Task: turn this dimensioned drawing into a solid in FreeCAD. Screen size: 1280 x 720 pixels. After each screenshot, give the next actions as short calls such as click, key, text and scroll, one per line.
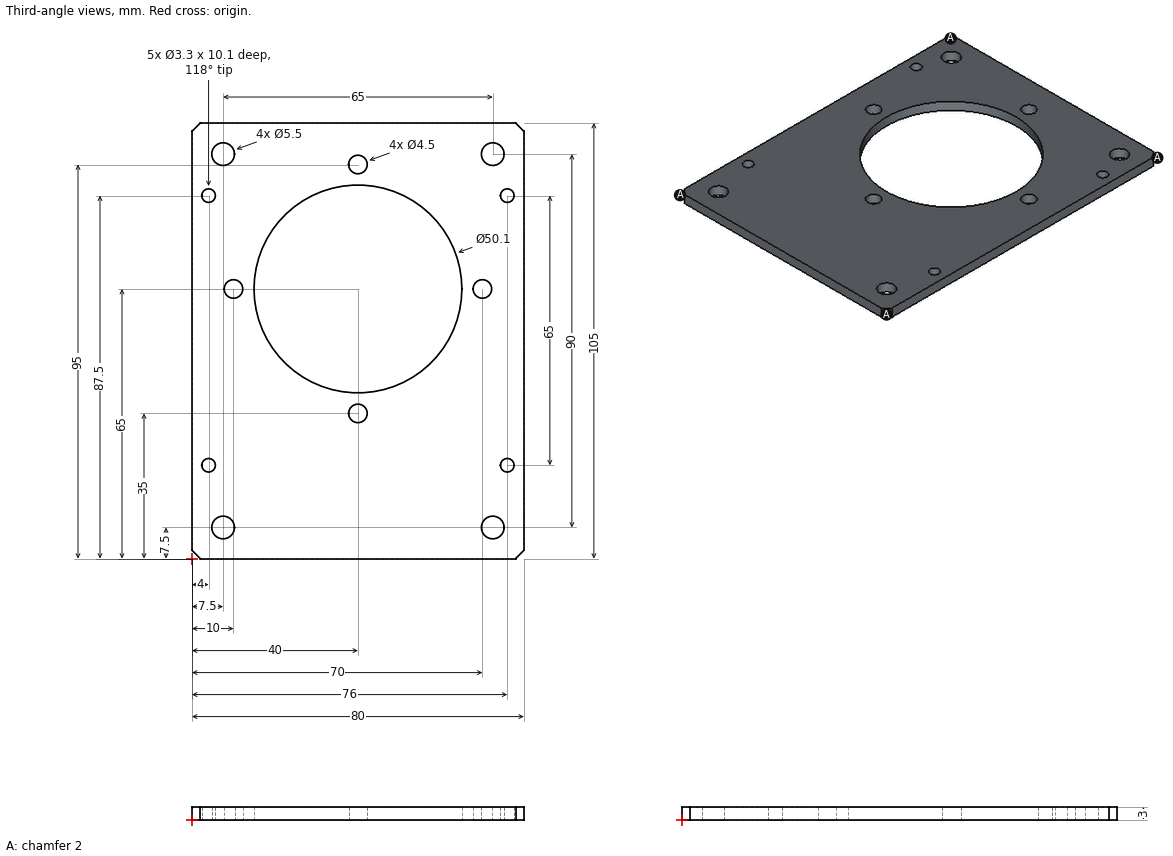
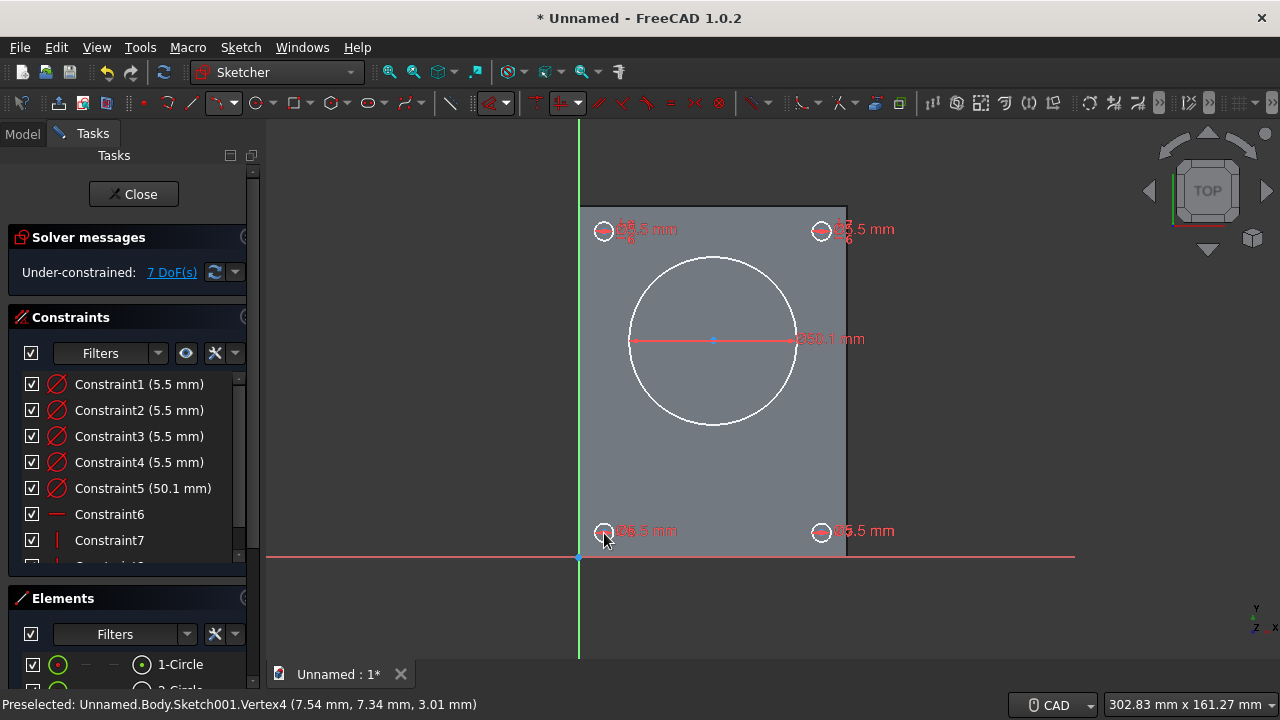
click(822, 533)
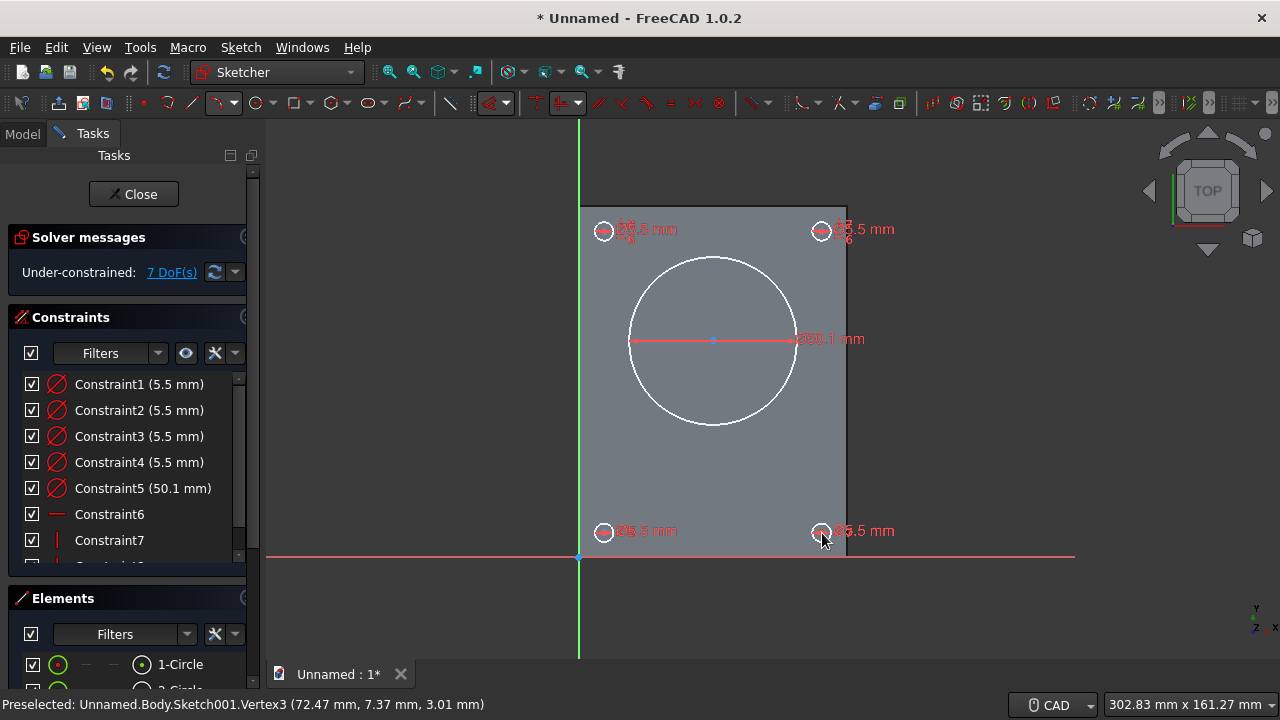
click(604, 533)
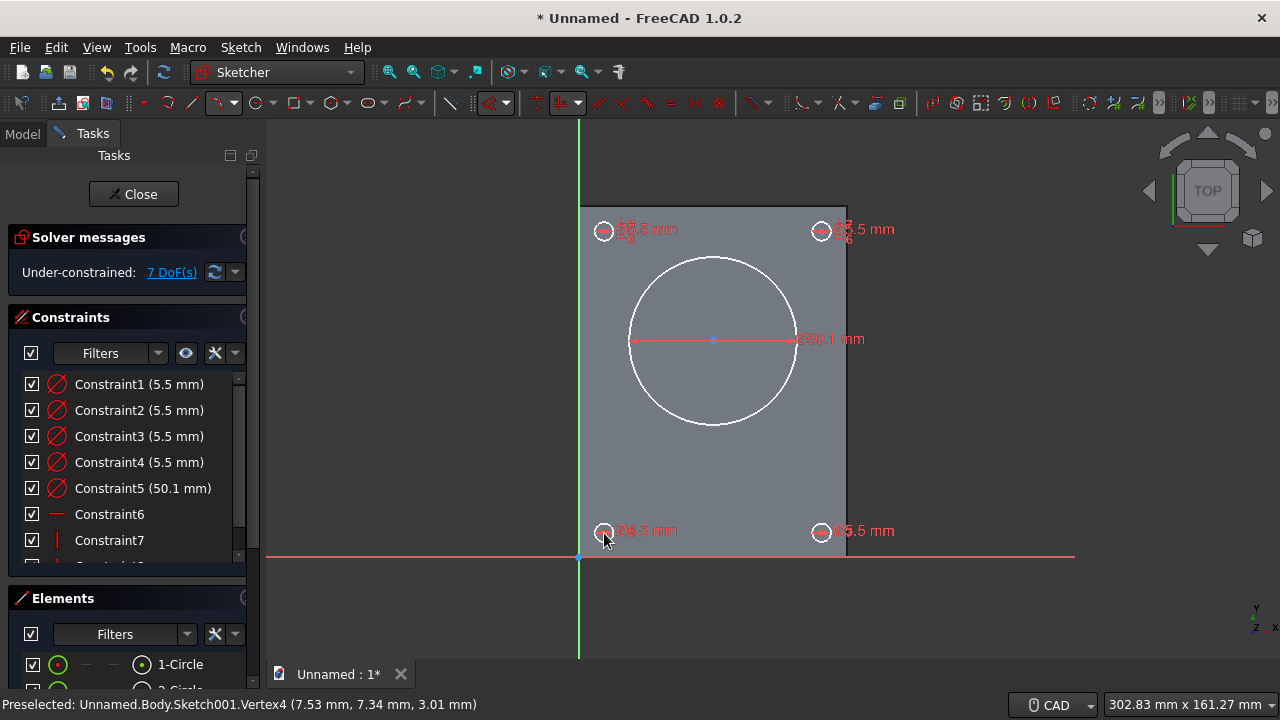
click(580, 104)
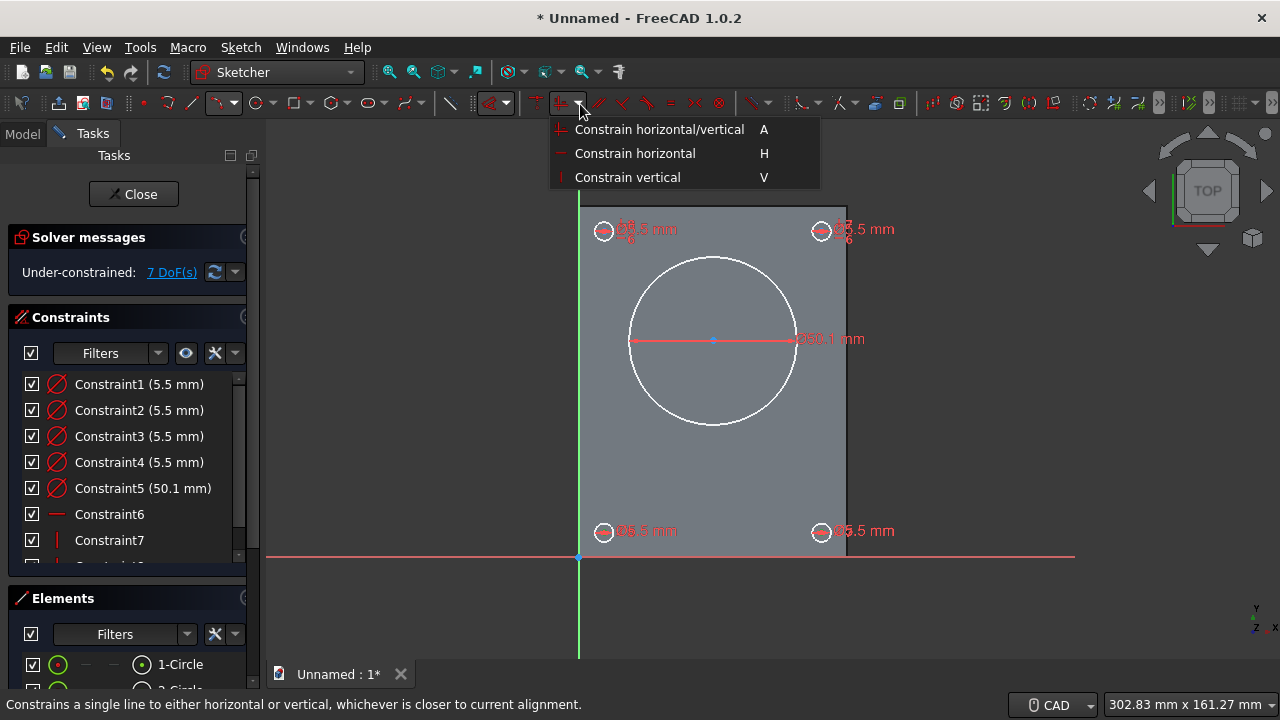
click(685, 153)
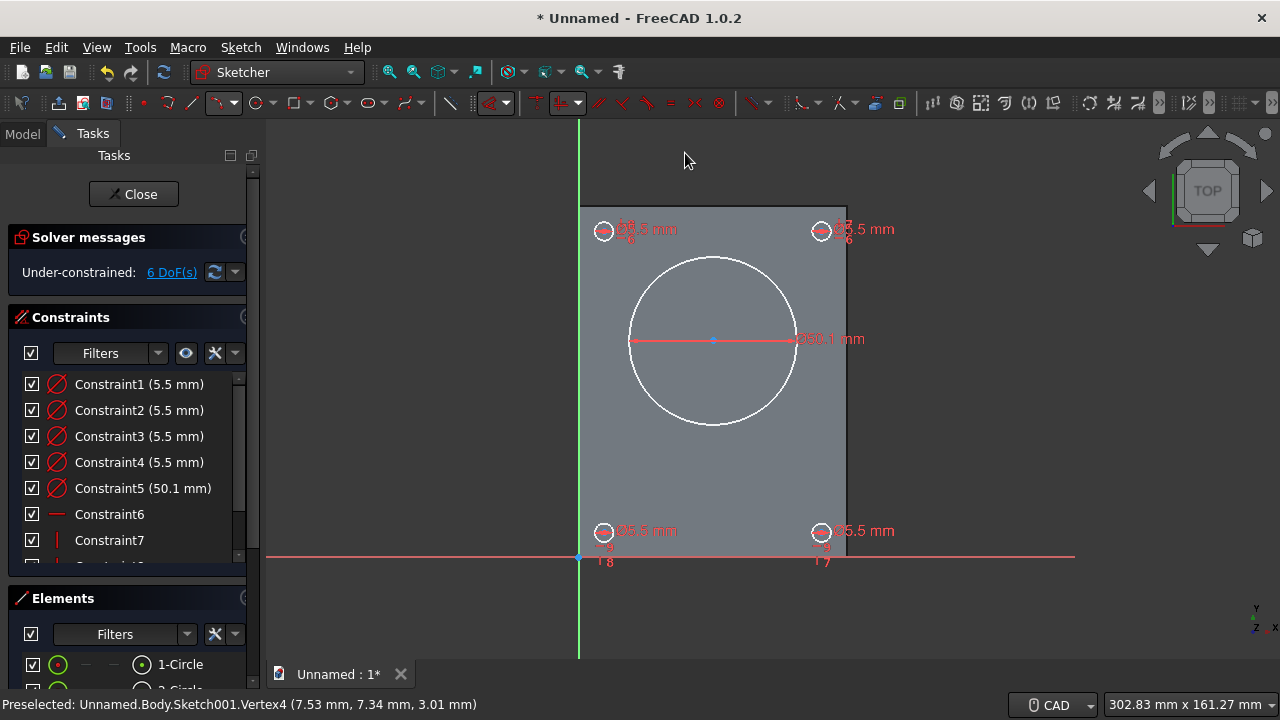
click(713, 341)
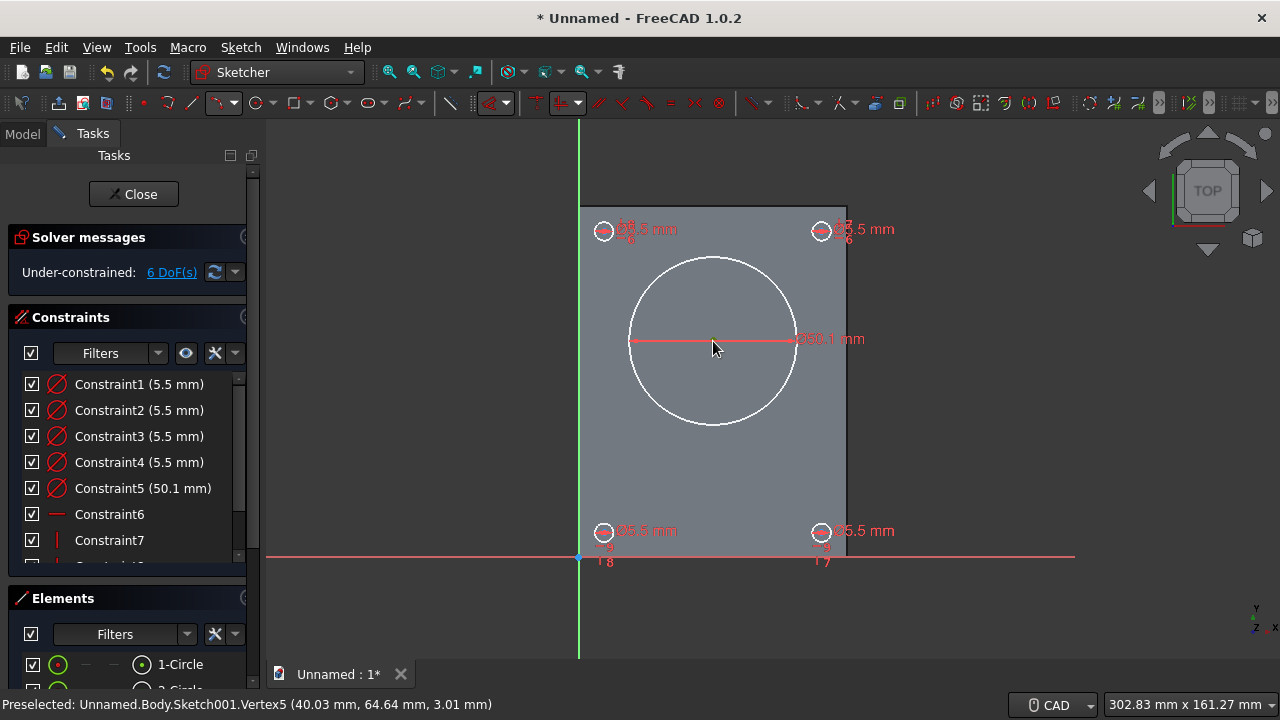
key(l)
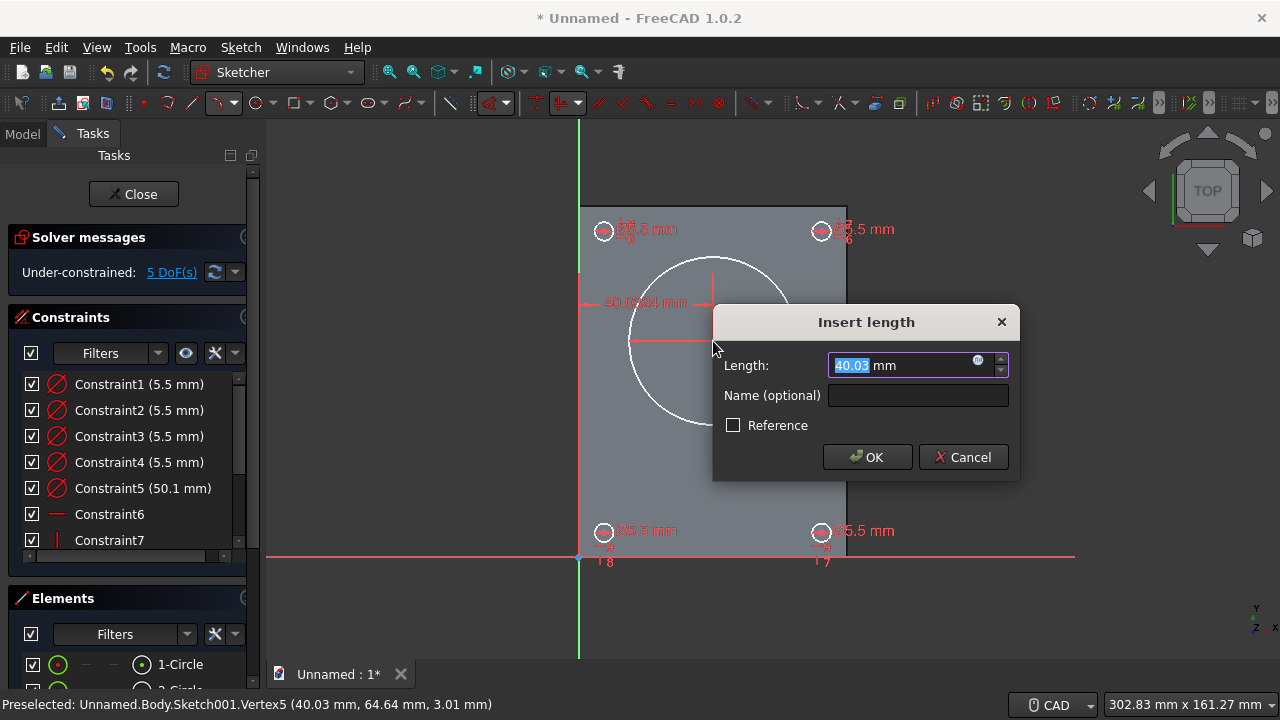
text(40)
key(Return)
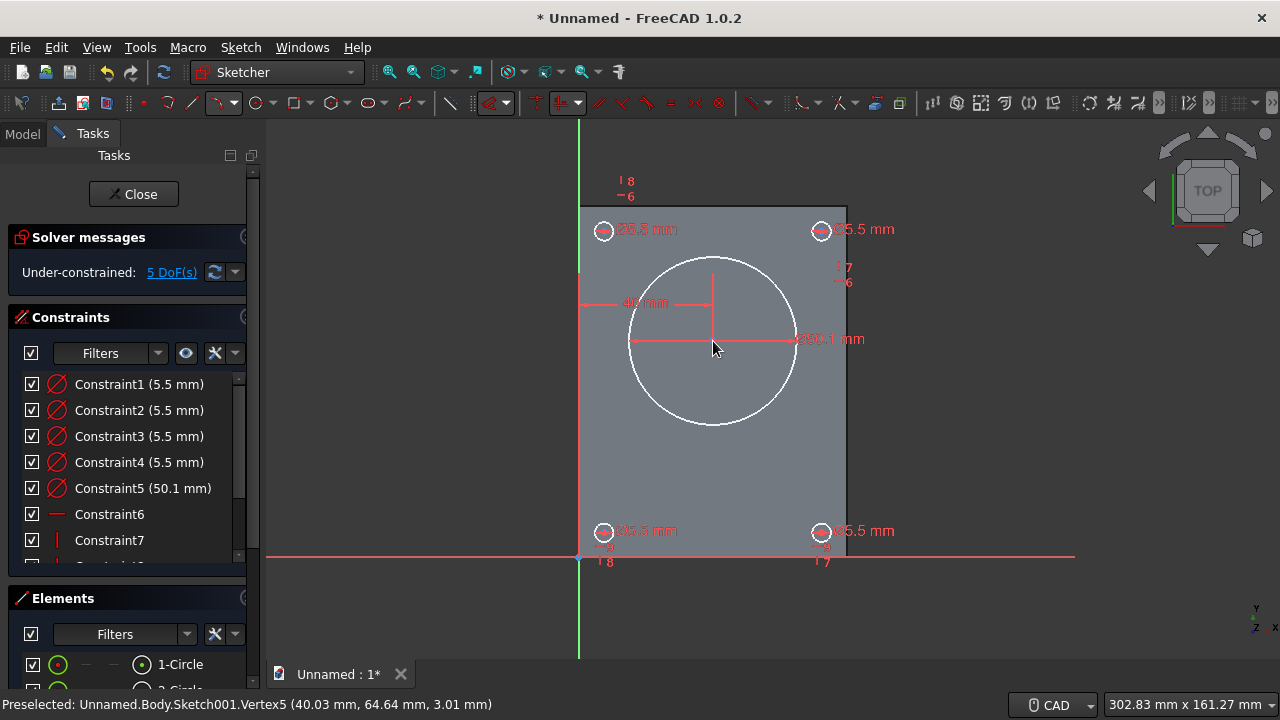
click(713, 341)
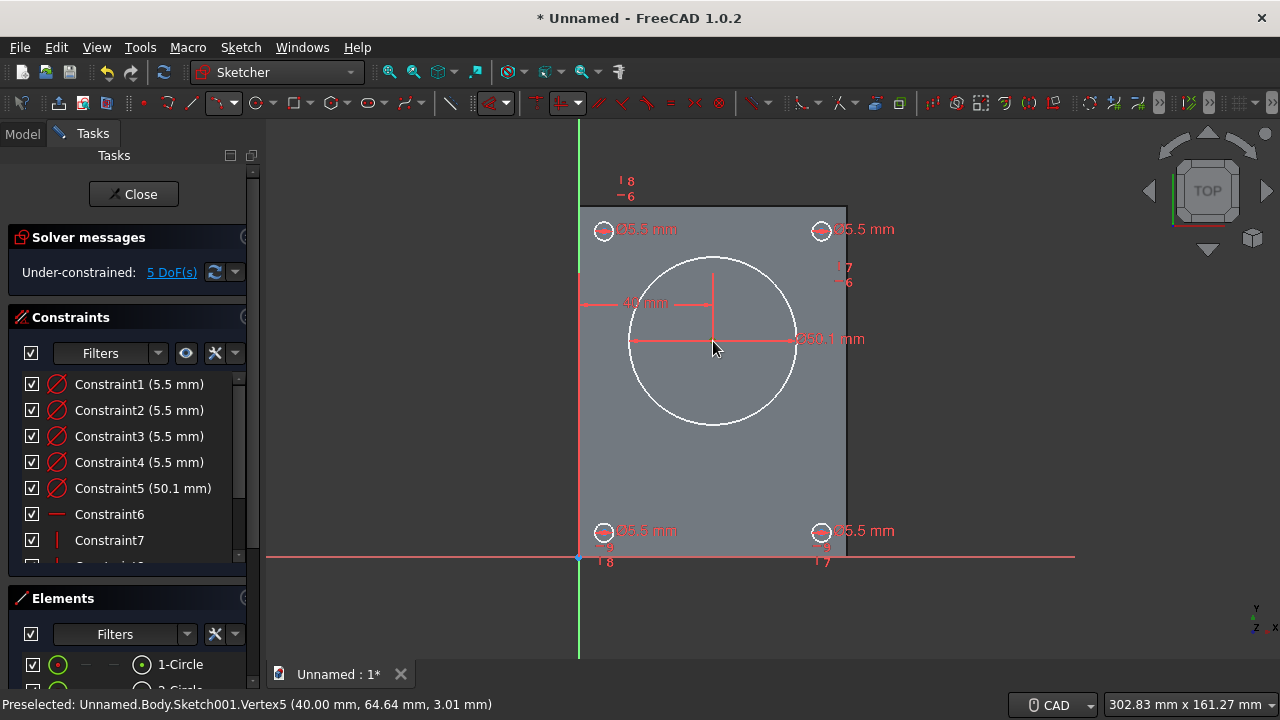
click(508, 104)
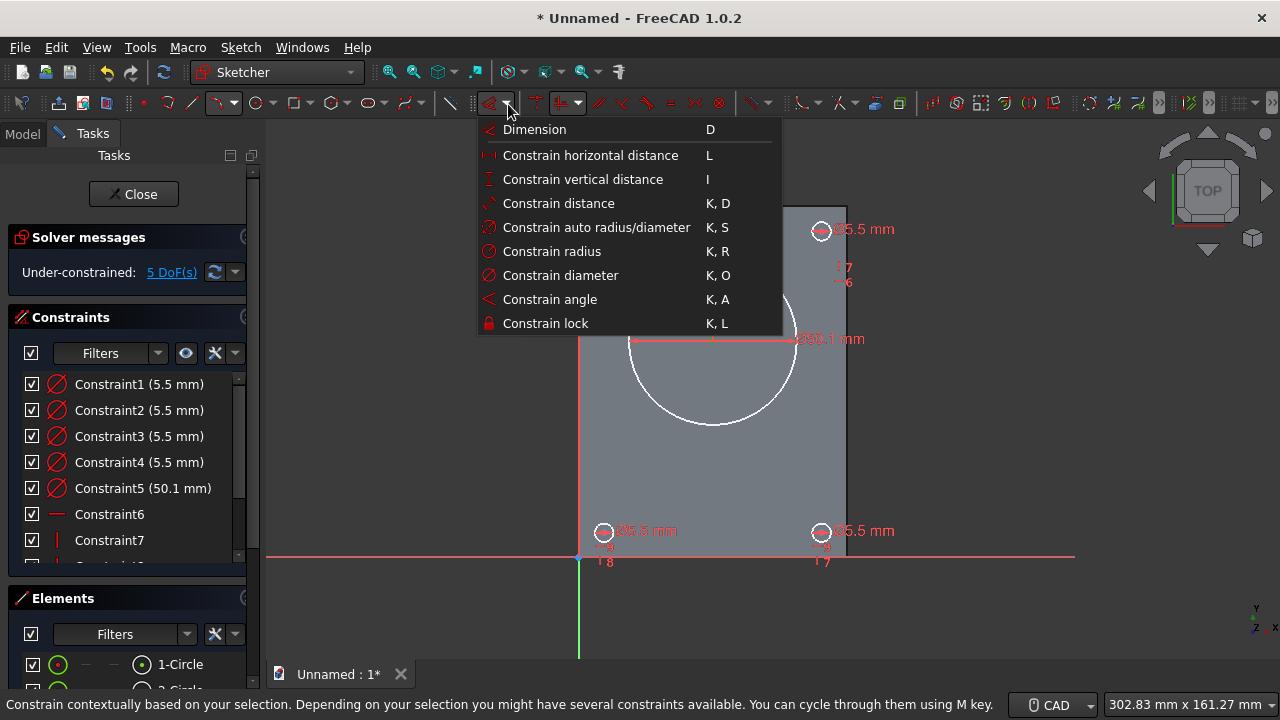
click(630, 179)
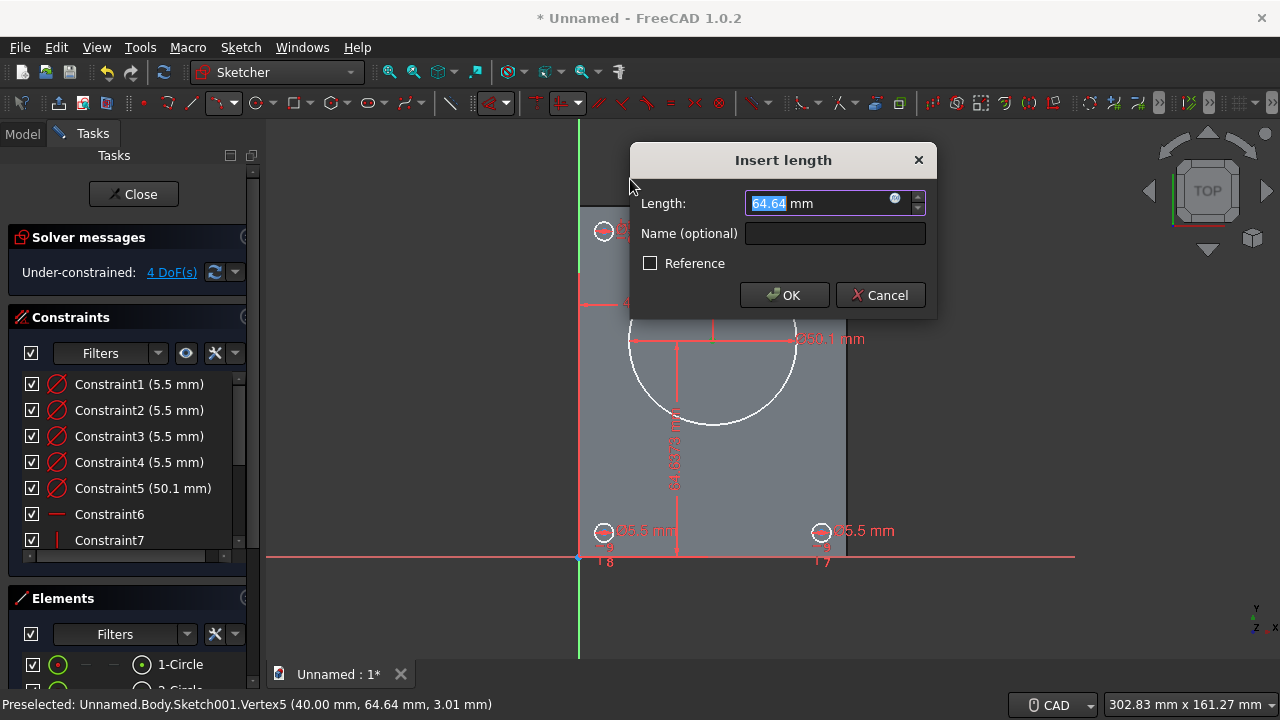
text(65)
key(Return)